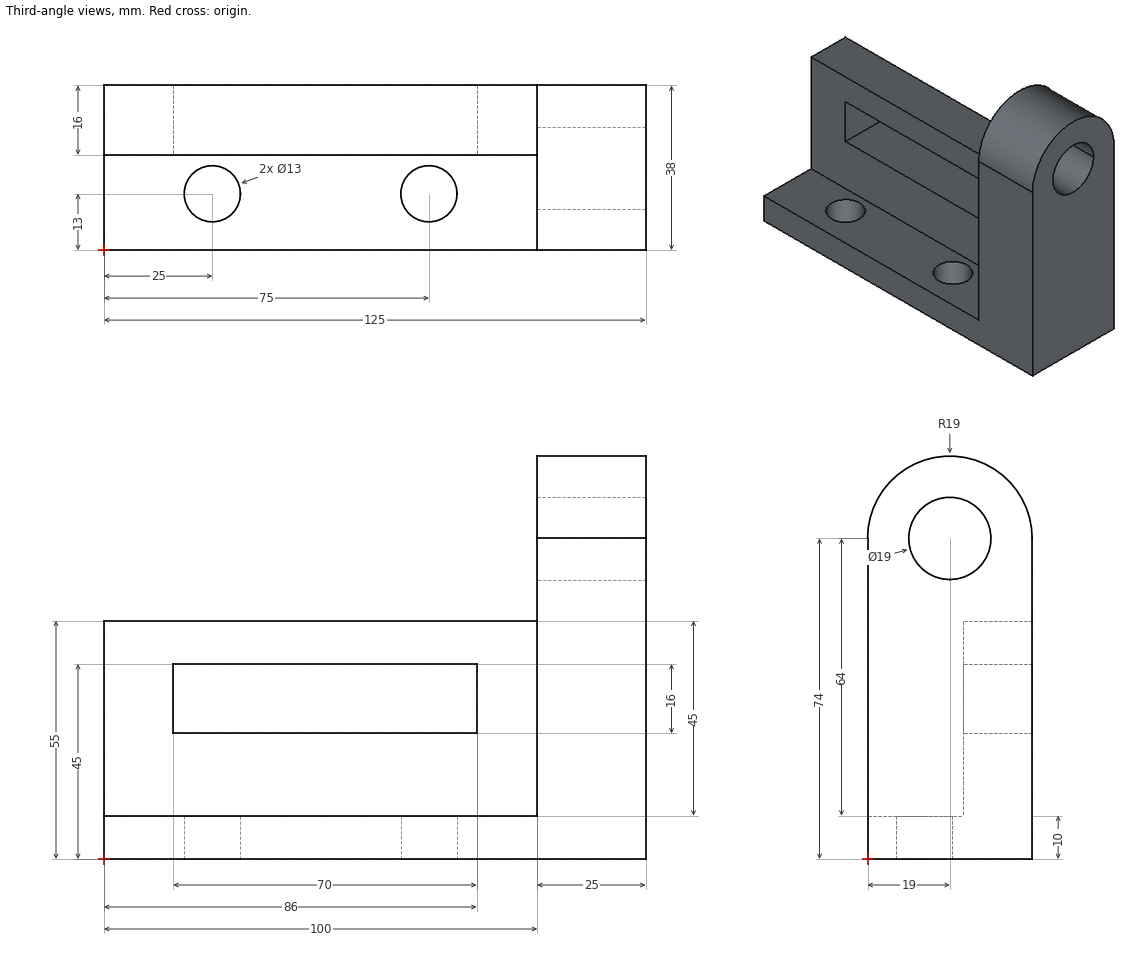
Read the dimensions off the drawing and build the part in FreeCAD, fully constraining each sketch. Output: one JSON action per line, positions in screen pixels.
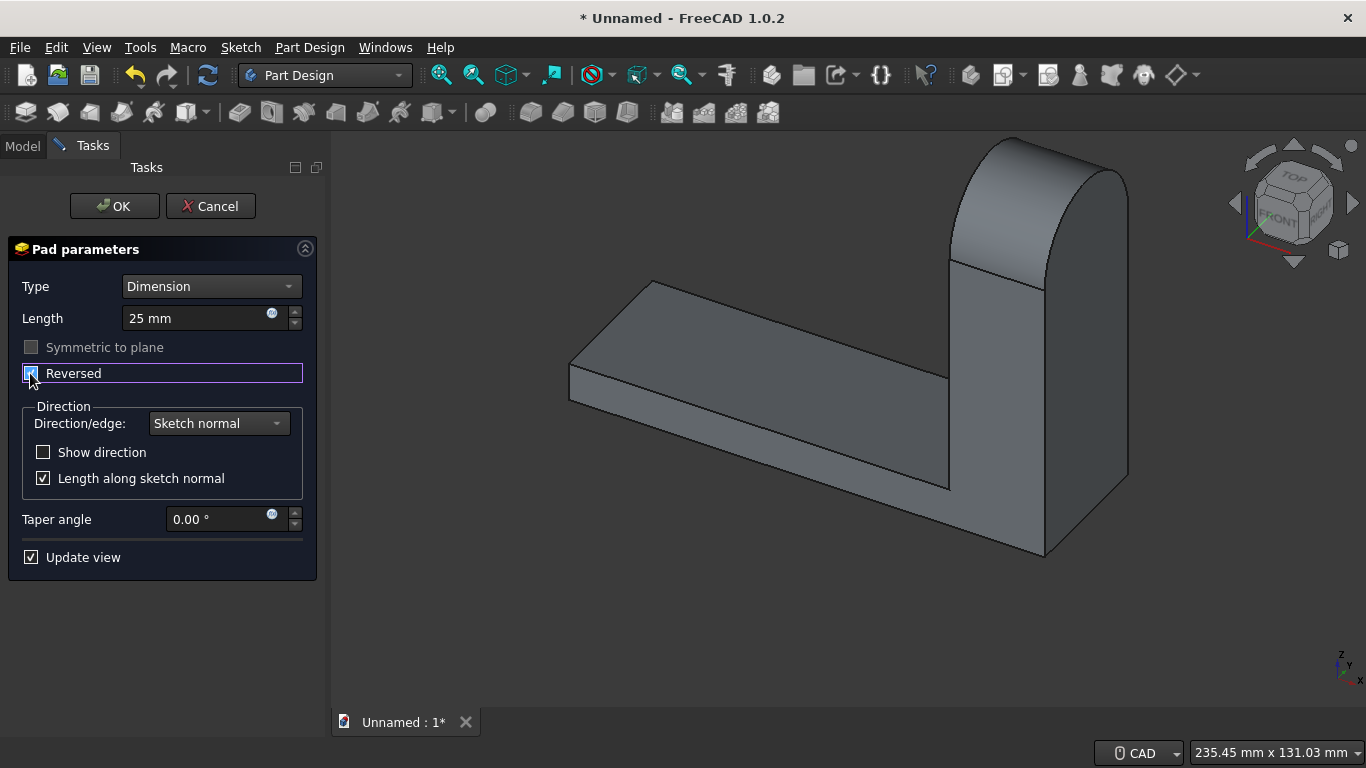
{"action": "left_click", "coordinate": [115, 206]}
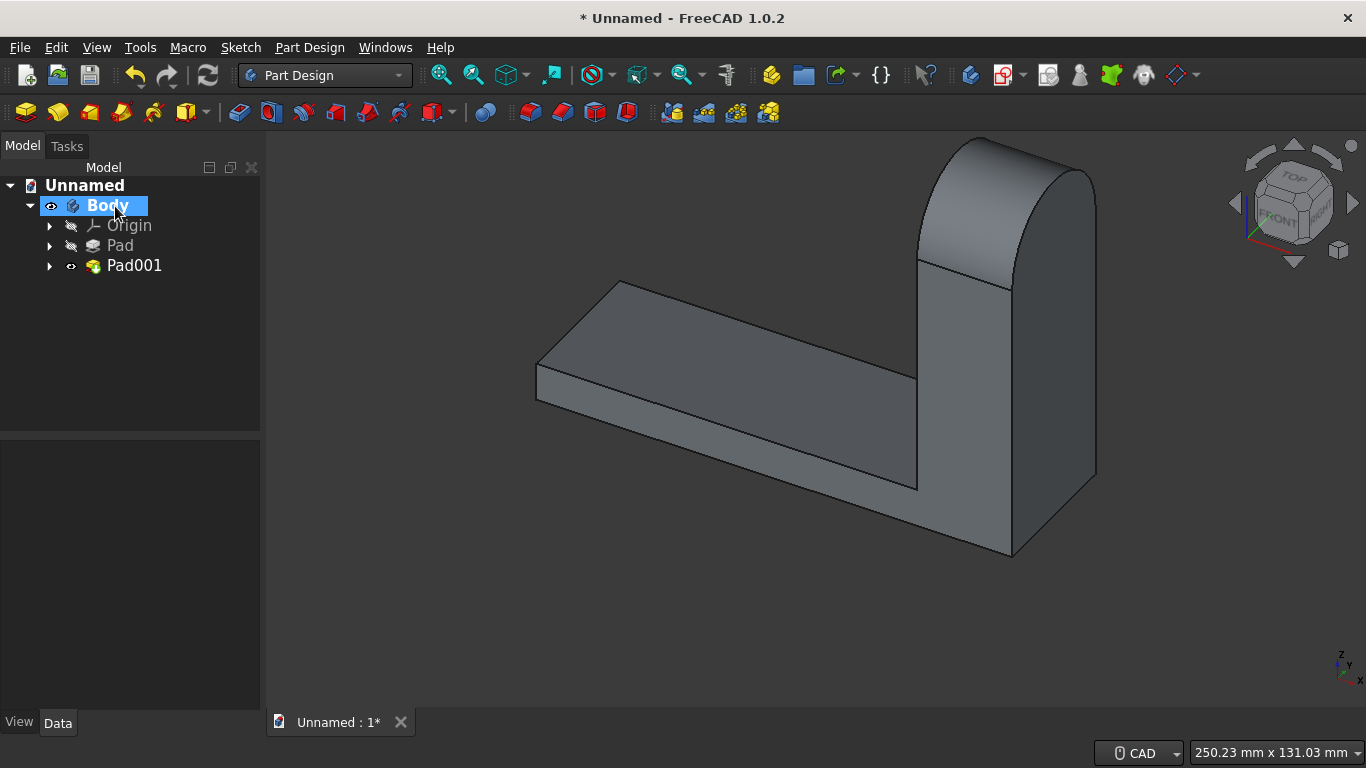
{"action": "left_click", "coordinate": [442, 76]}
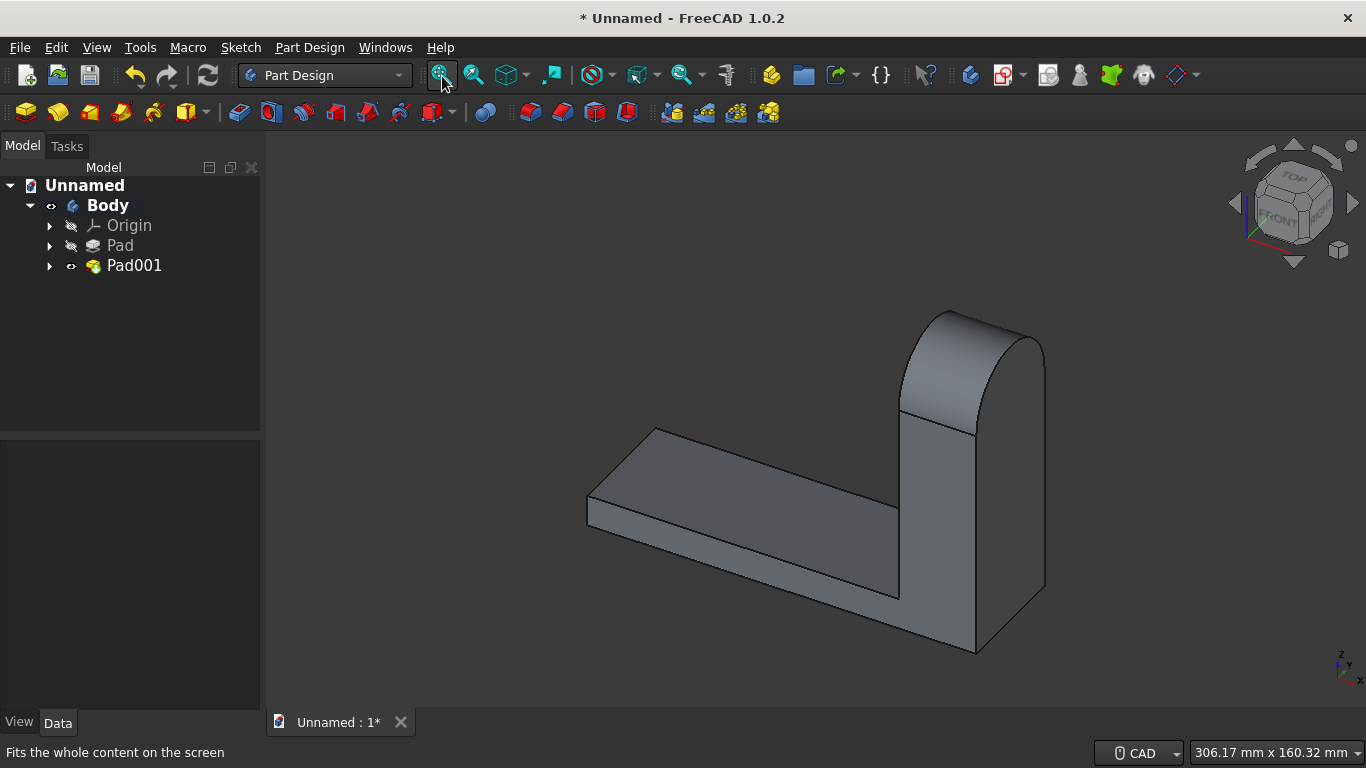
{"action": "left_click", "coordinate": [1010, 404]}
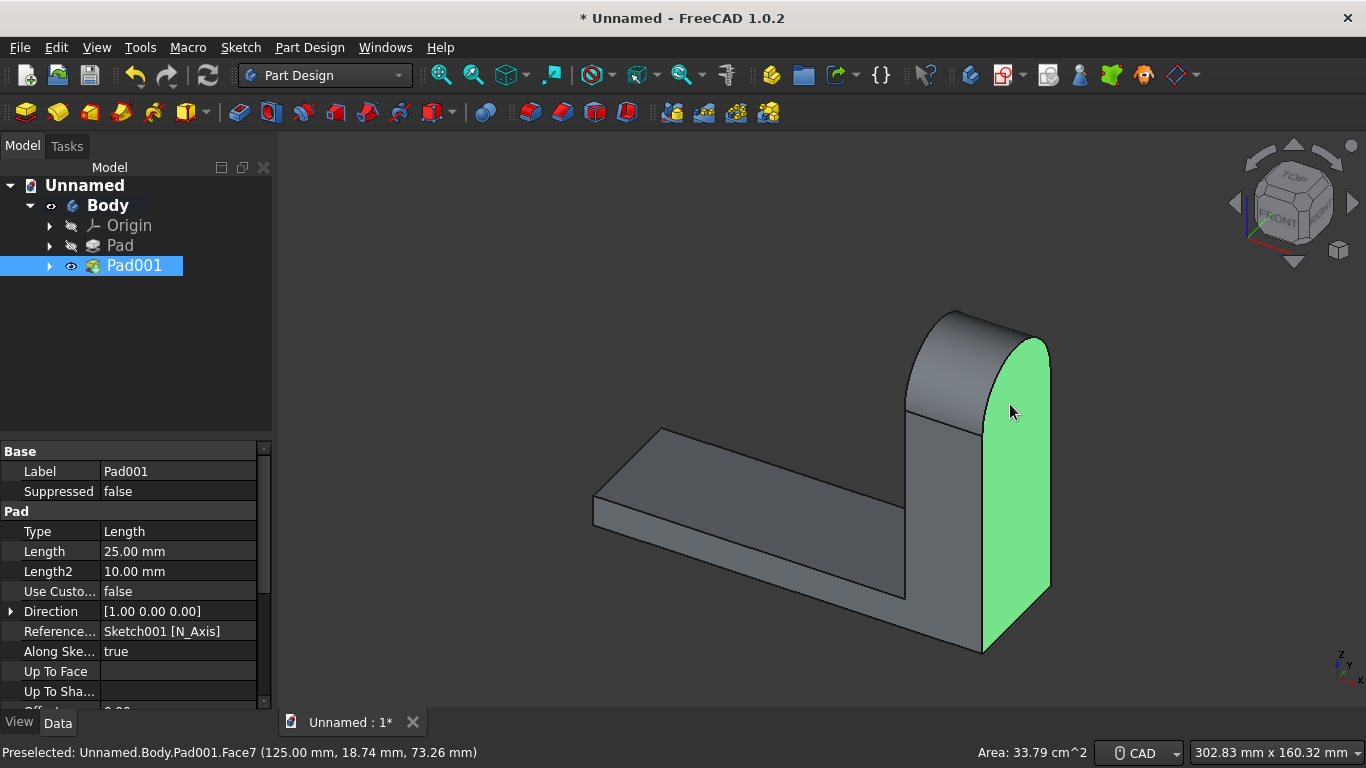
{"action": "left_click", "coordinate": [1004, 76]}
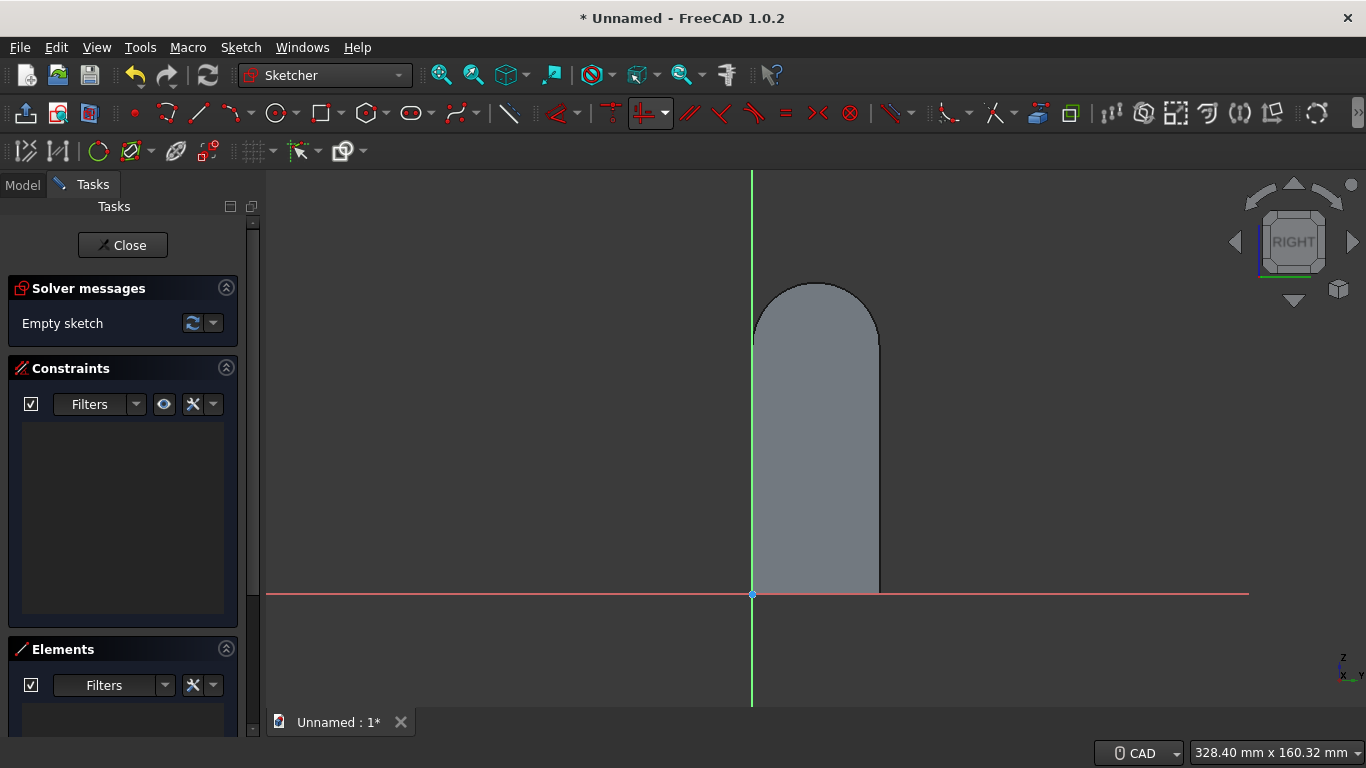
{"action": "scroll", "coordinate": [833, 323], "scroll_direction": "up", "scroll_amount": 8}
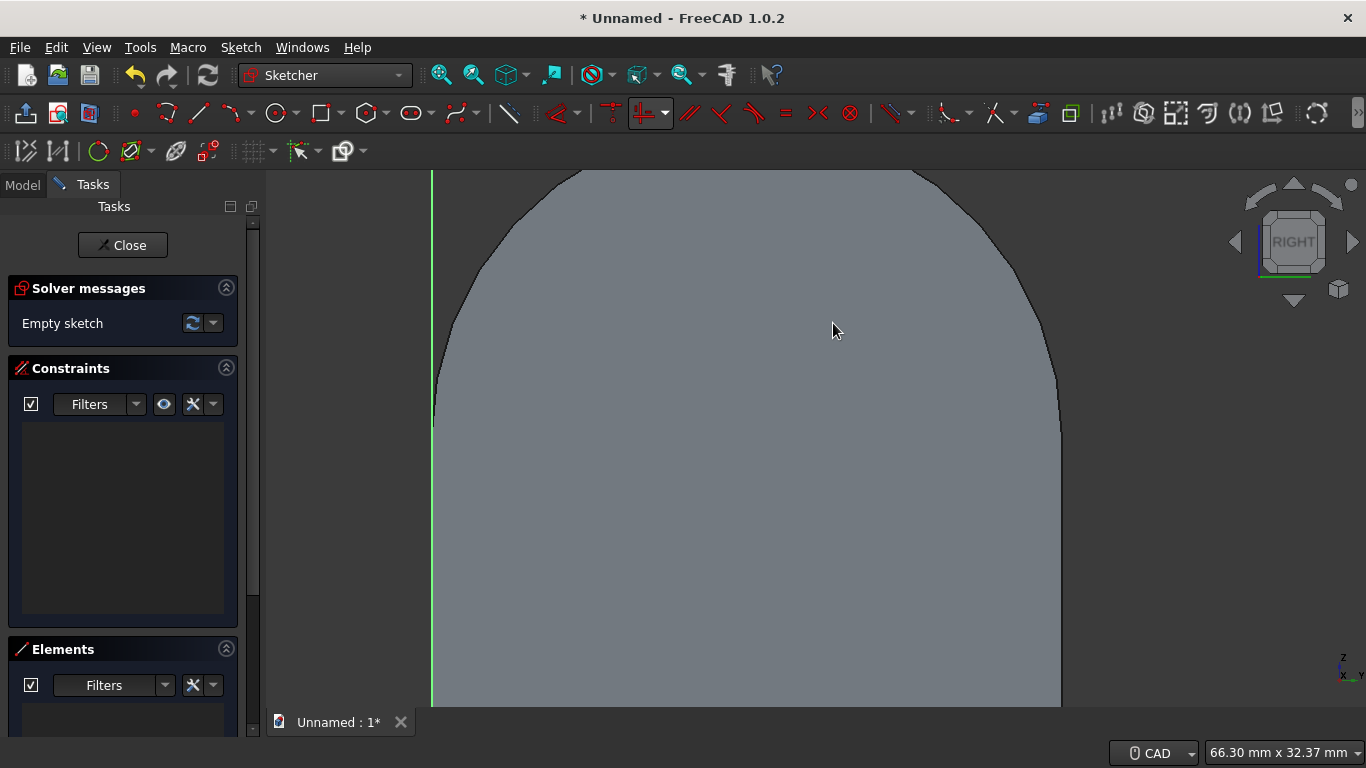
{"action": "left_click", "coordinate": [276, 114]}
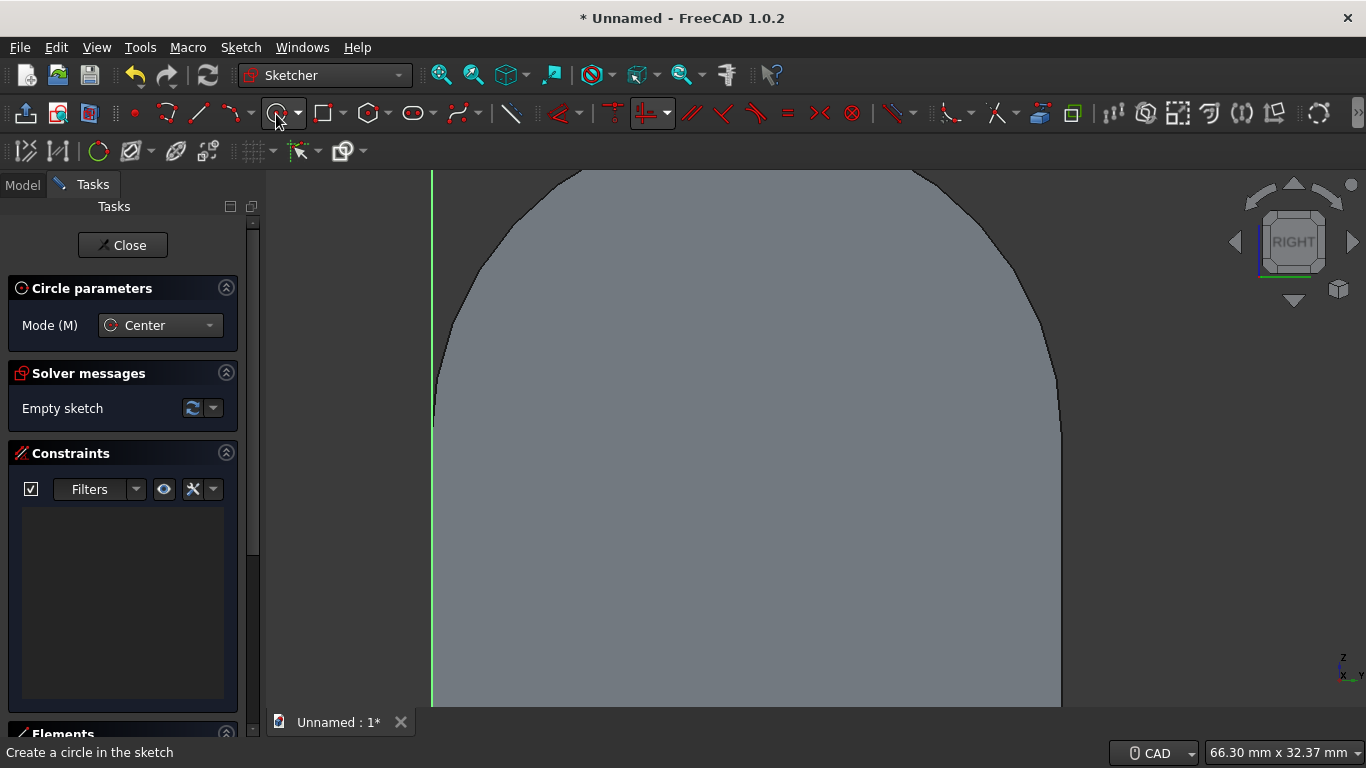
{"action": "left_click", "coordinate": [747, 437]}
{"action": "left_click", "coordinate": [858, 326]}
{"action": "key", "text": "Escape"}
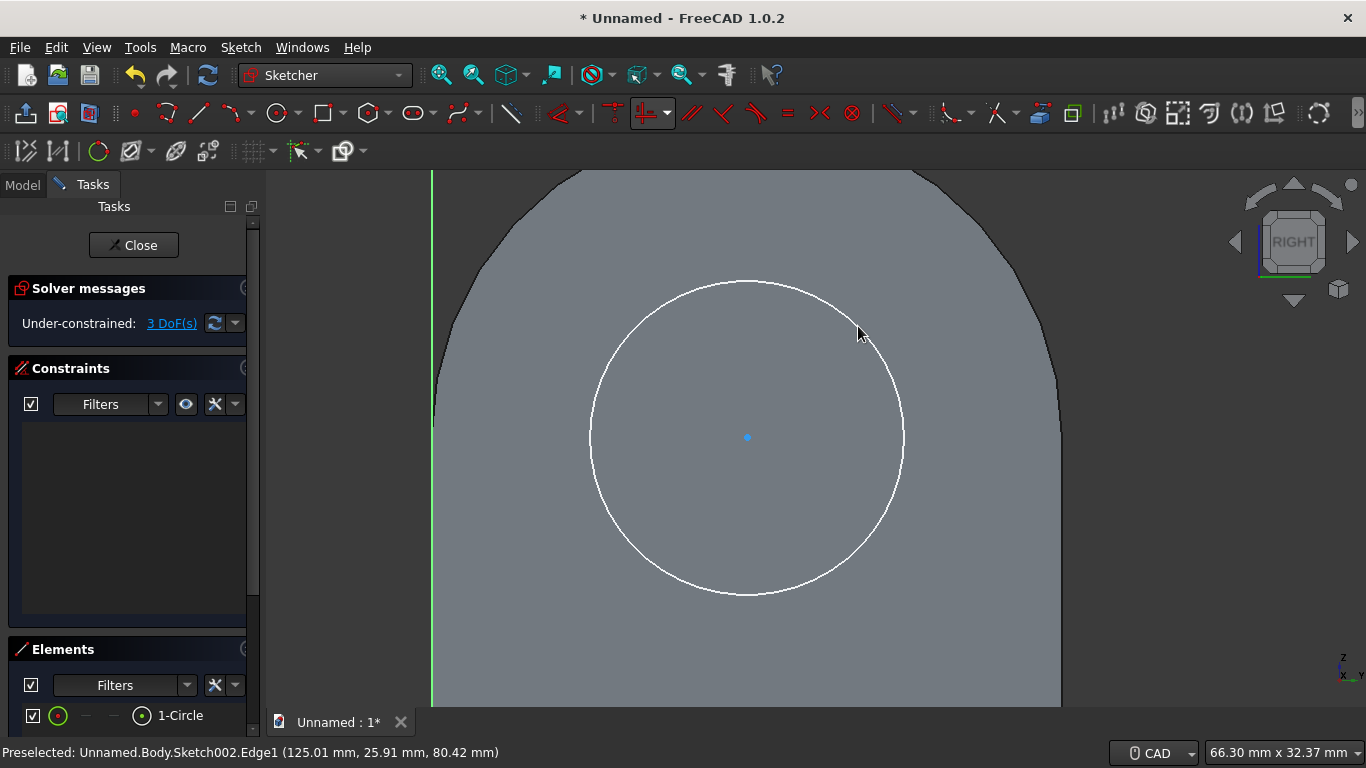
{"action": "left_click", "coordinate": [558, 114]}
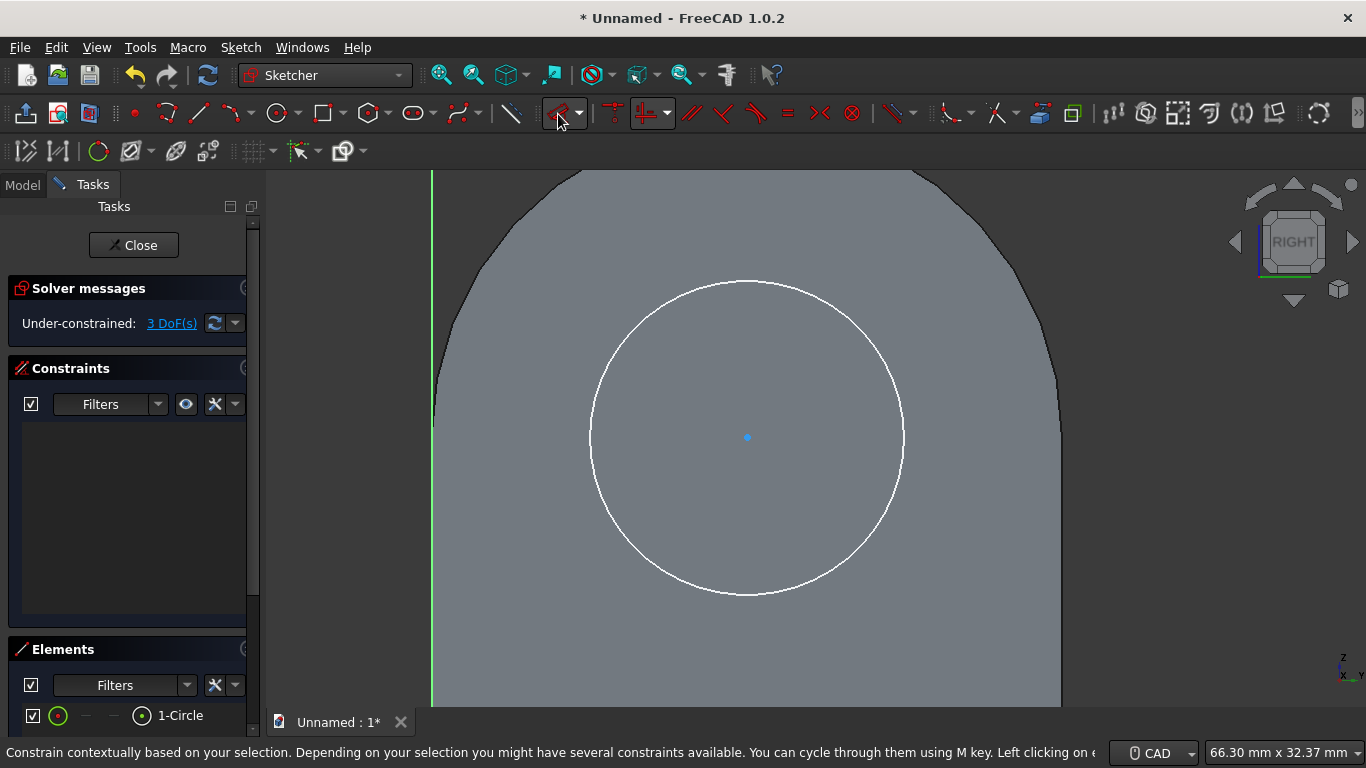
{"action": "left_click", "coordinate": [858, 327]}
{"action": "left_click", "coordinate": [881, 304]}